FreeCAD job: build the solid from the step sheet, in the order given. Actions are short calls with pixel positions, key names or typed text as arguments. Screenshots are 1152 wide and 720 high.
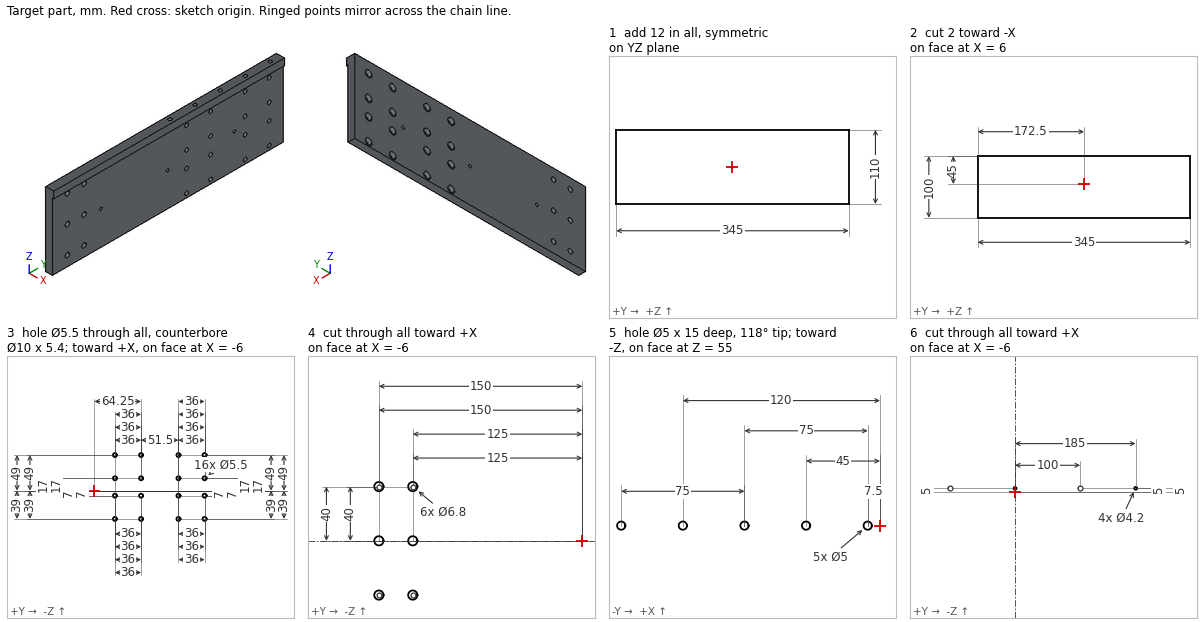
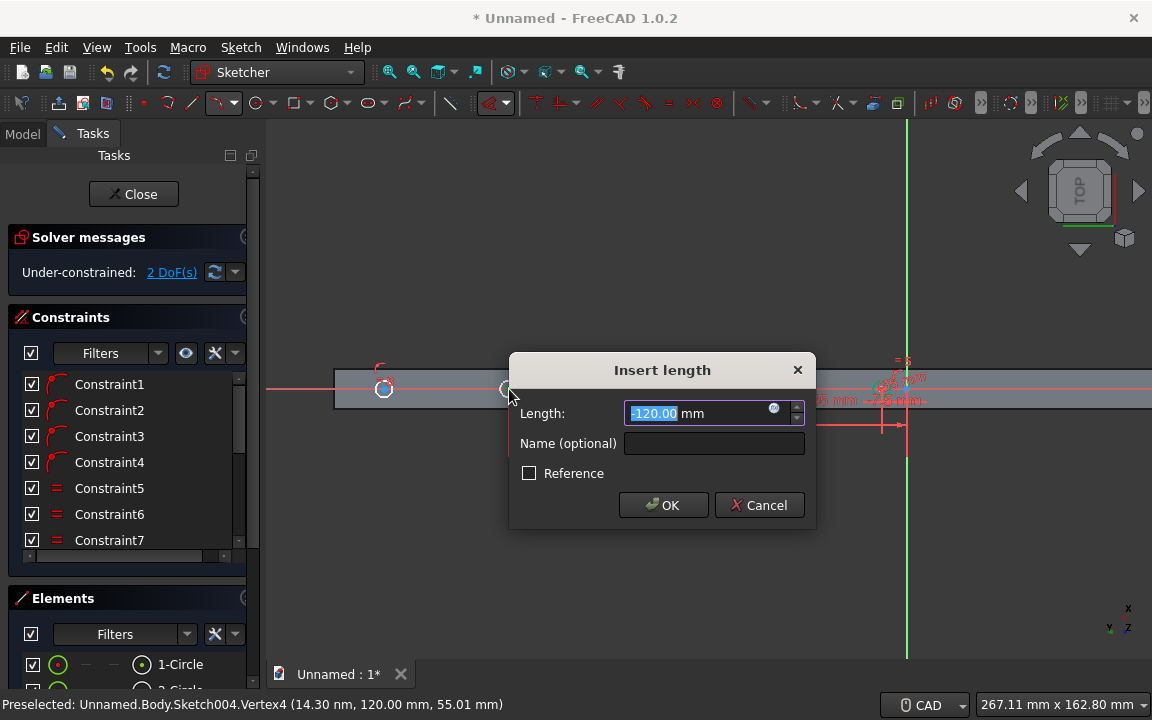
text(-120)
key(Return)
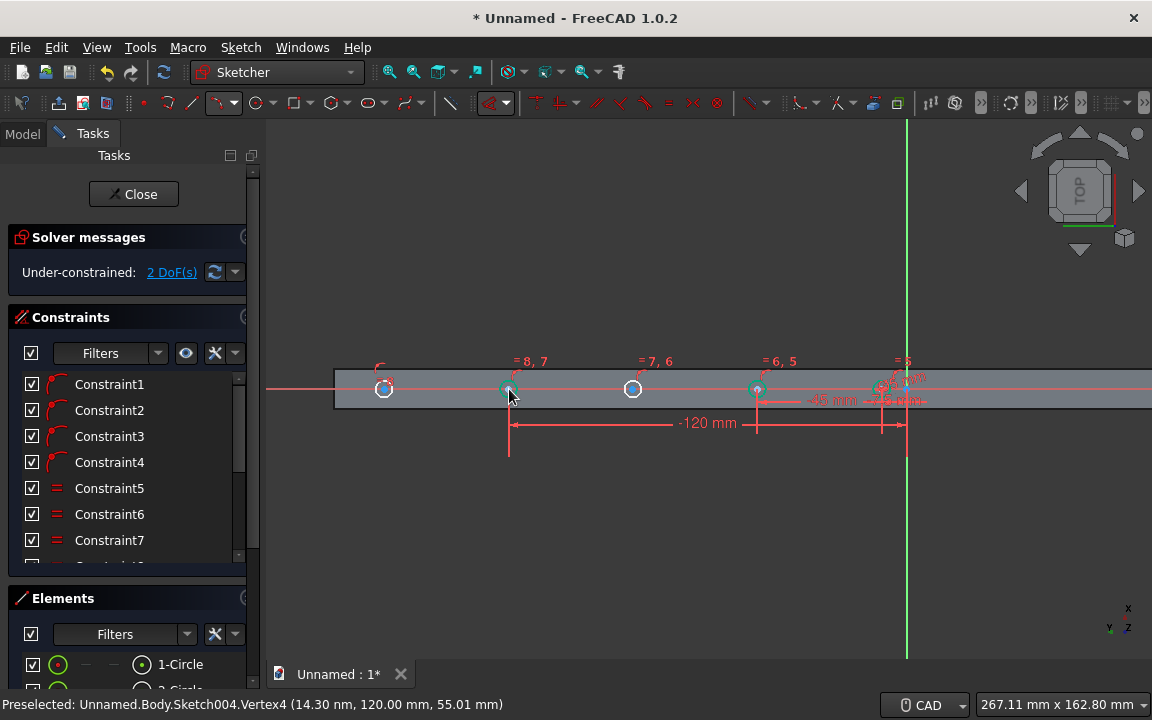
click(882, 389)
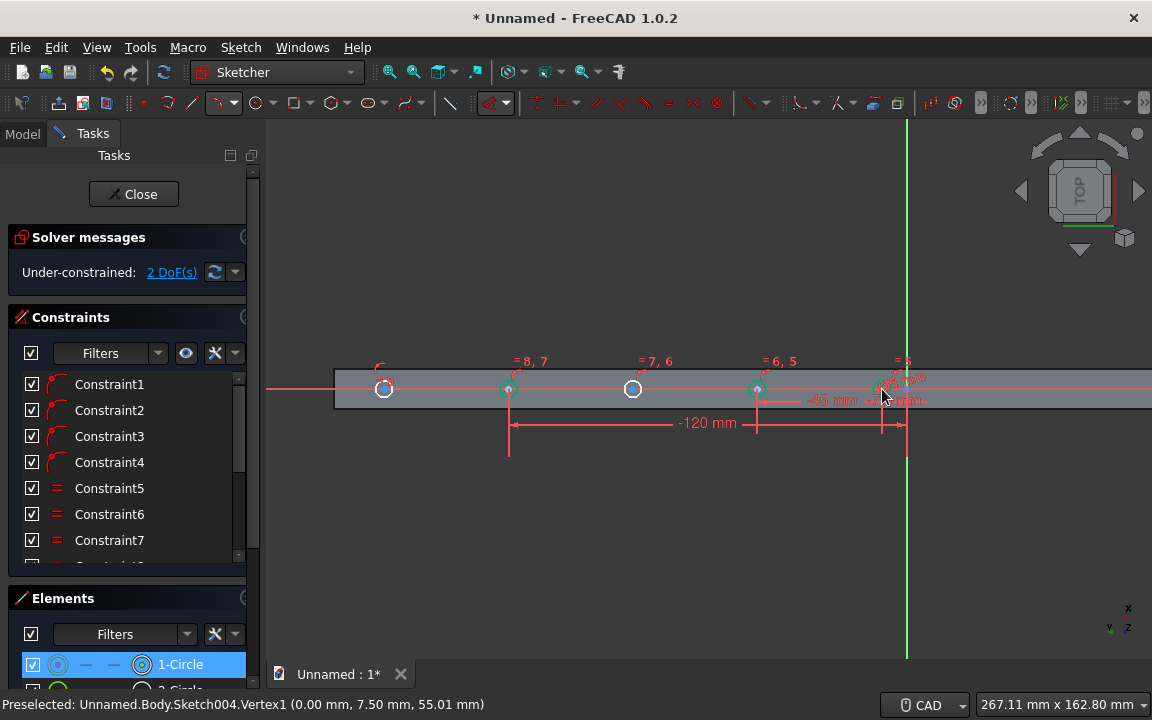
click(633, 389)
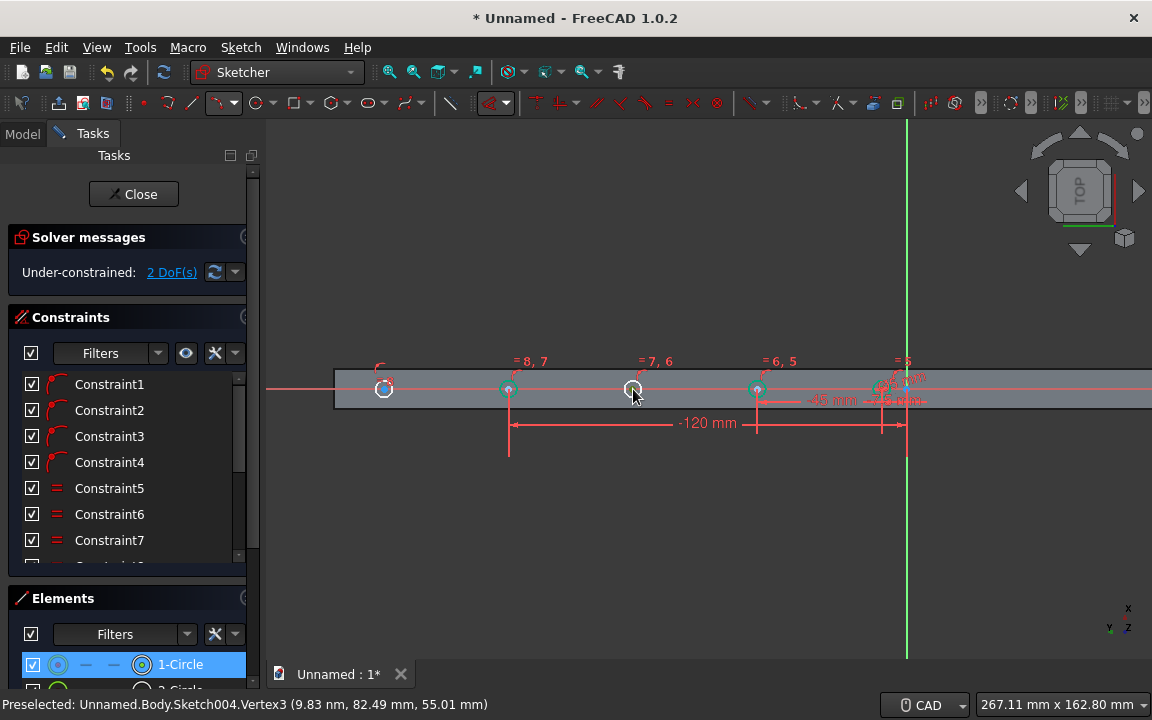
click(508, 104)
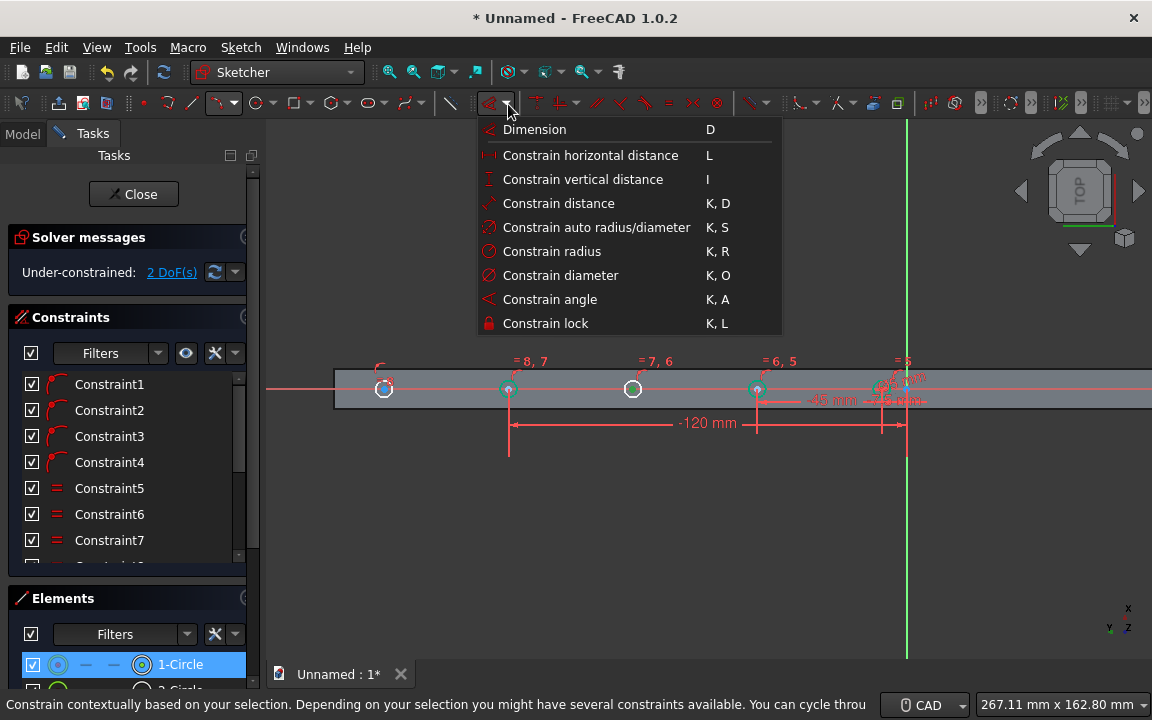
click(630, 155)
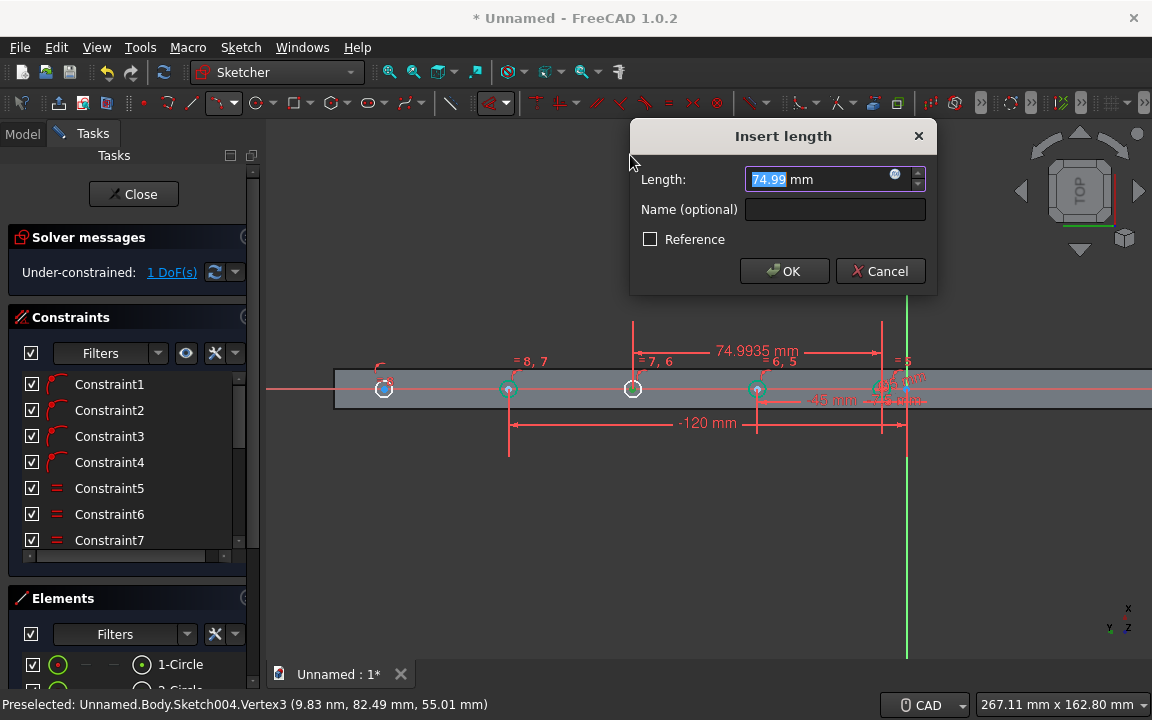
text(75)
key(Return)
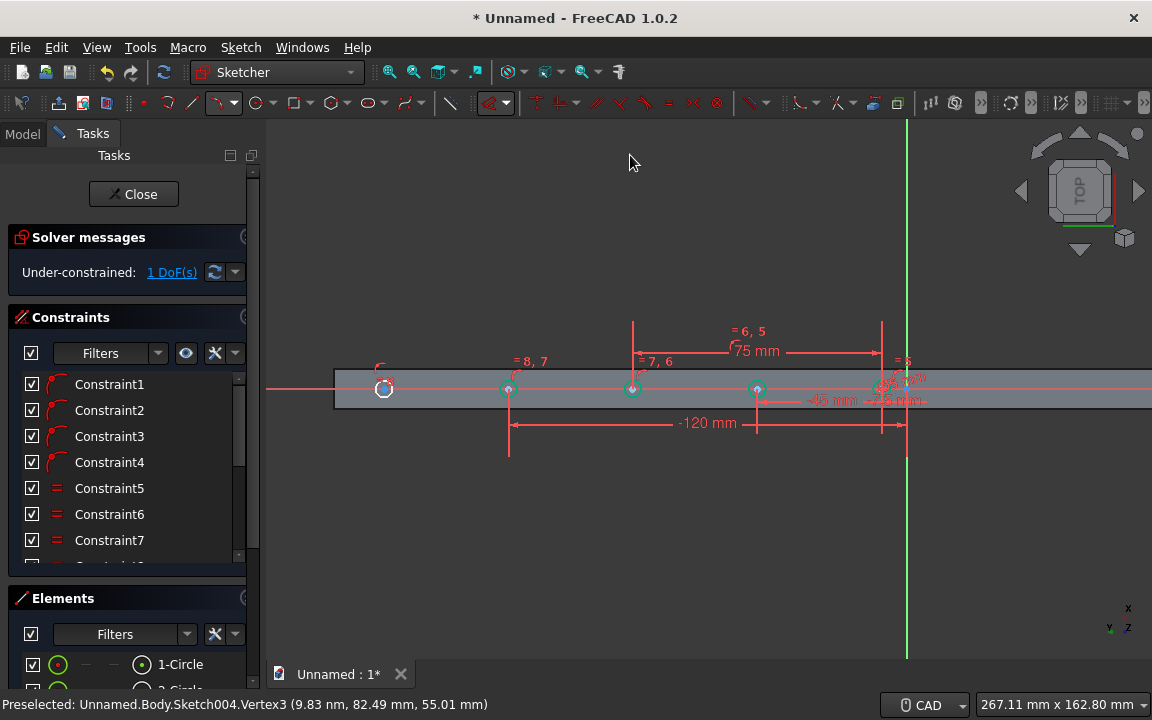
click(633, 389)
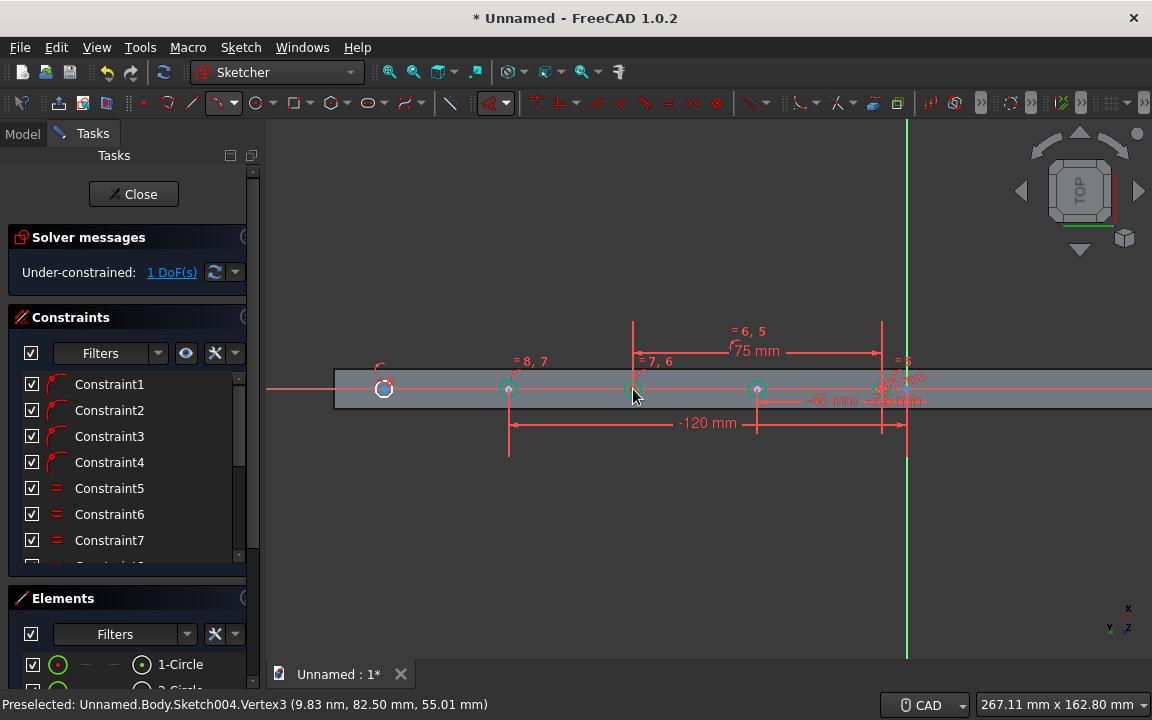
click(384, 389)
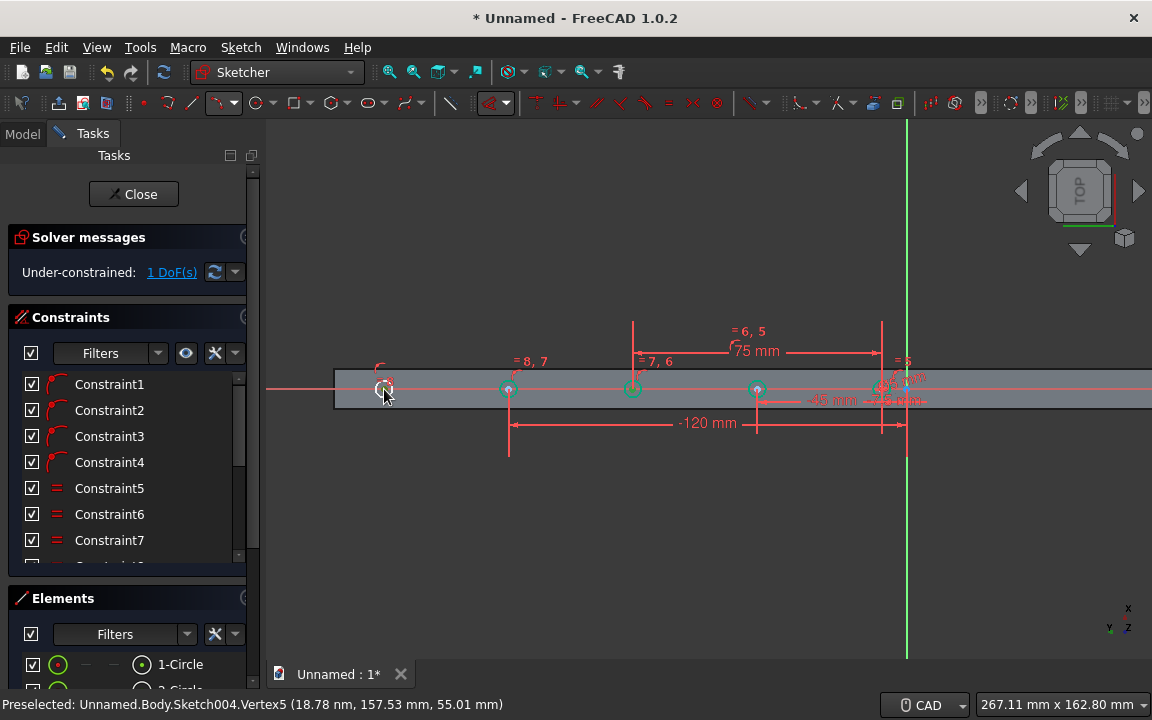
key(l)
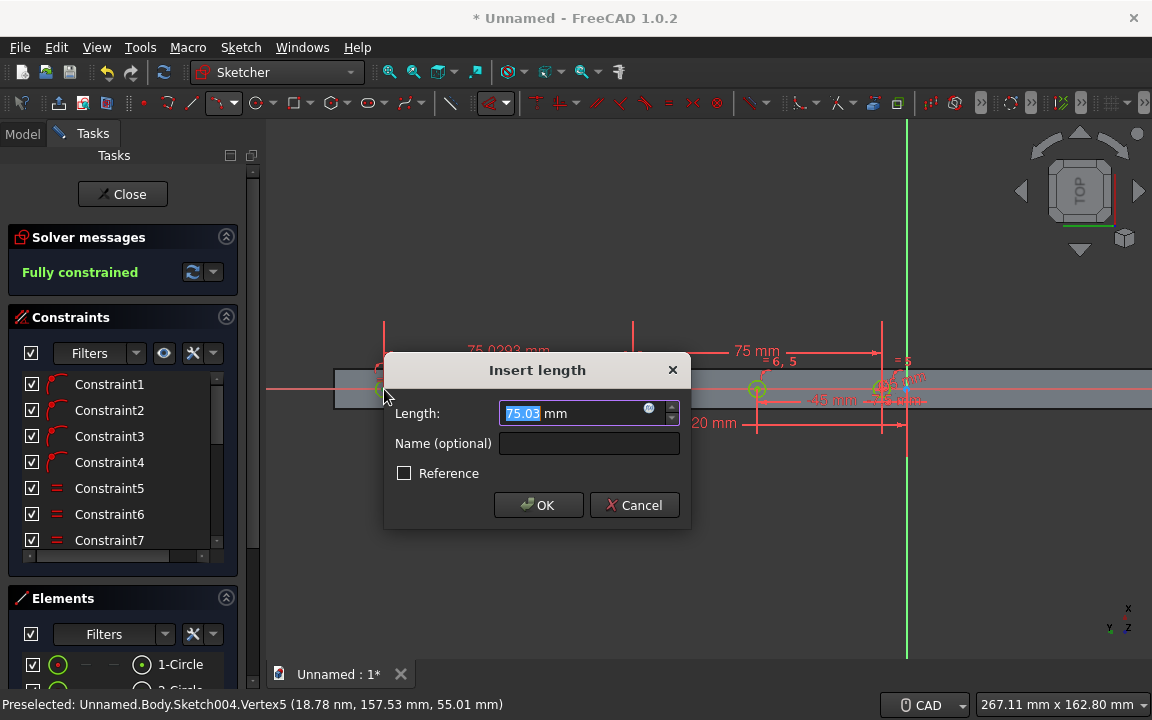
text(75)
key(Return)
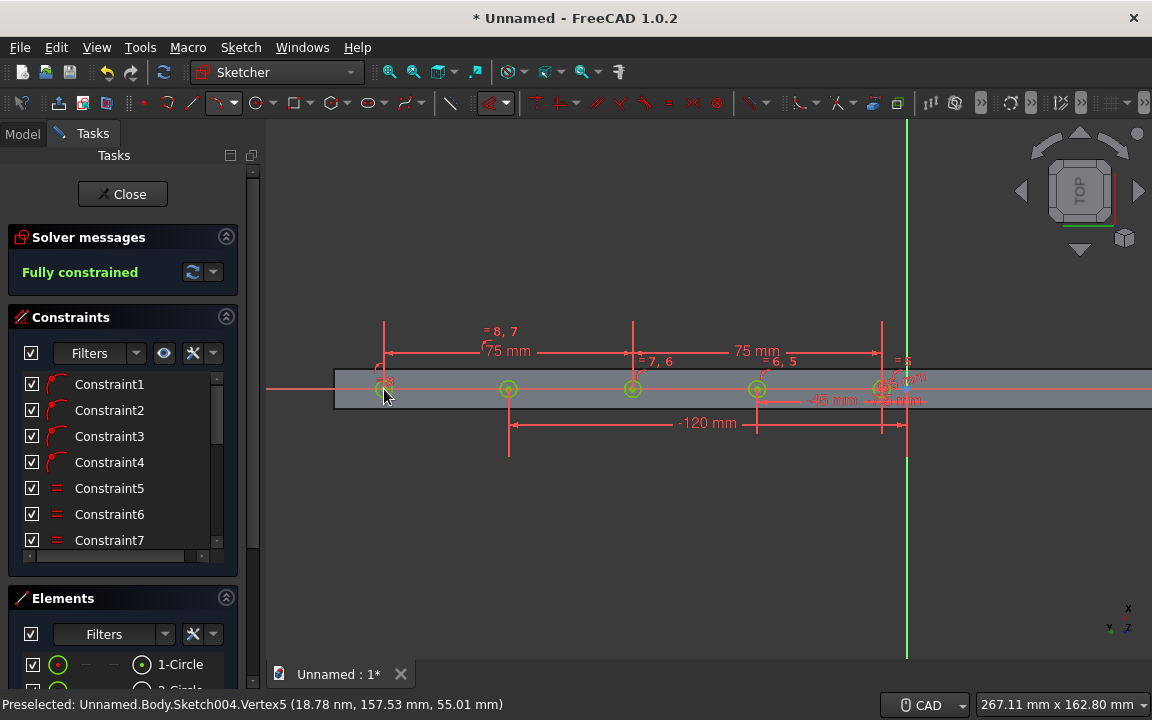
click(123, 194)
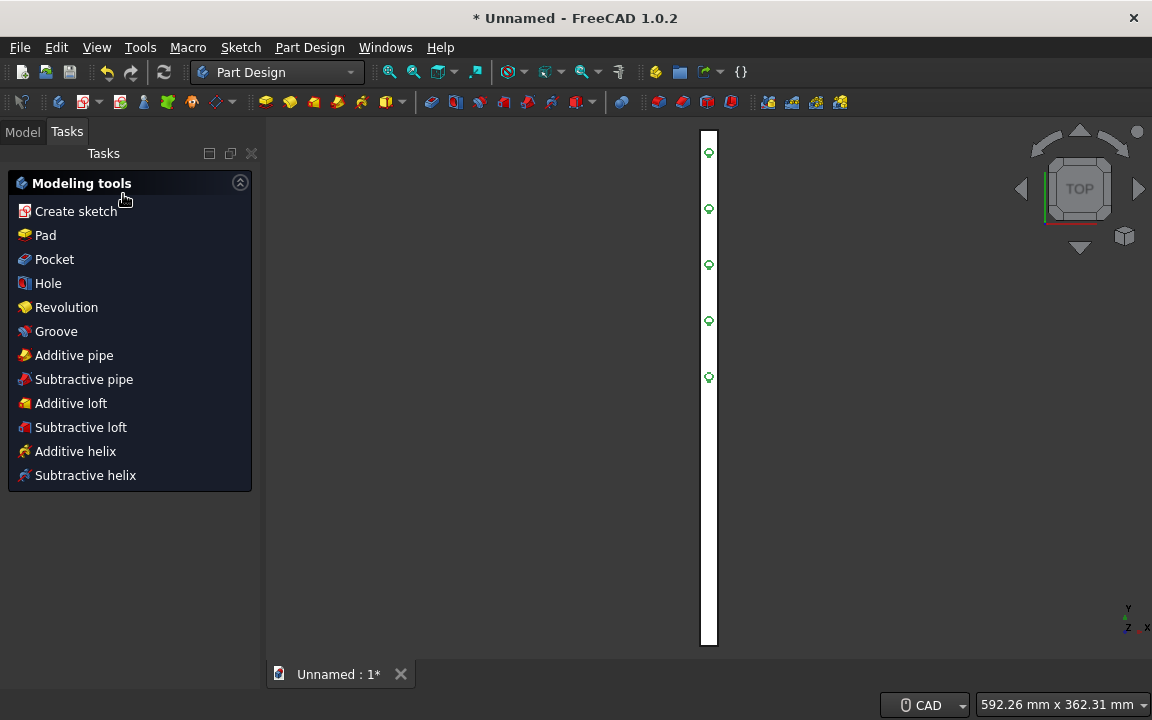
click(456, 102)